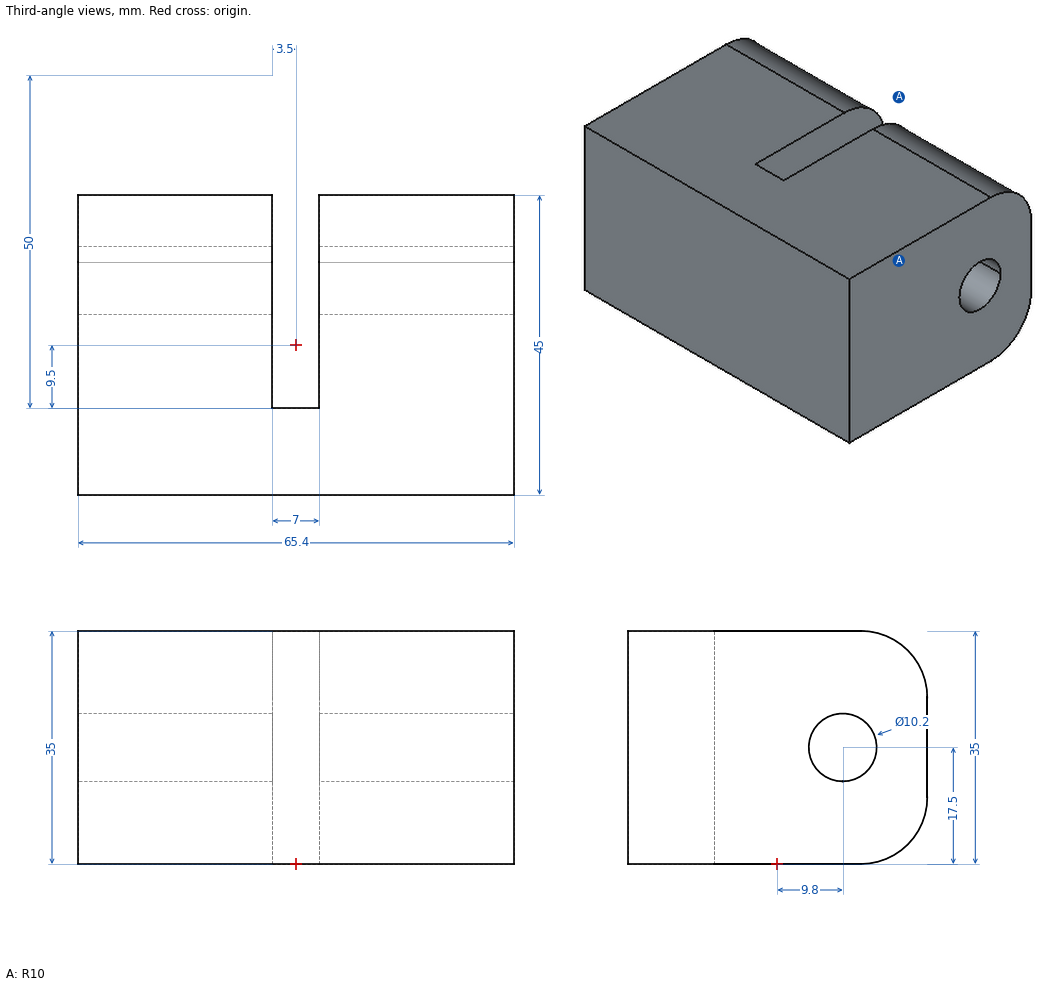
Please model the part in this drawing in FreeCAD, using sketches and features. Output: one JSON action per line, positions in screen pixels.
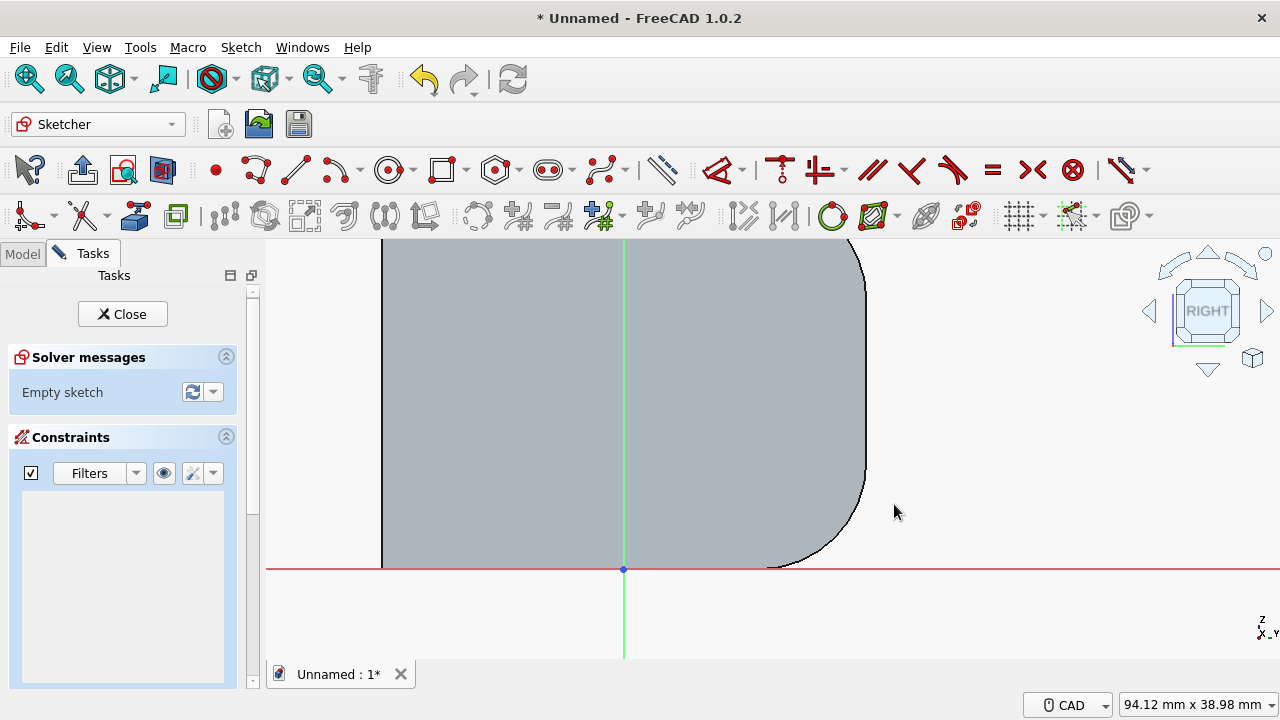
{"action": "left_click", "coordinate": [390, 170]}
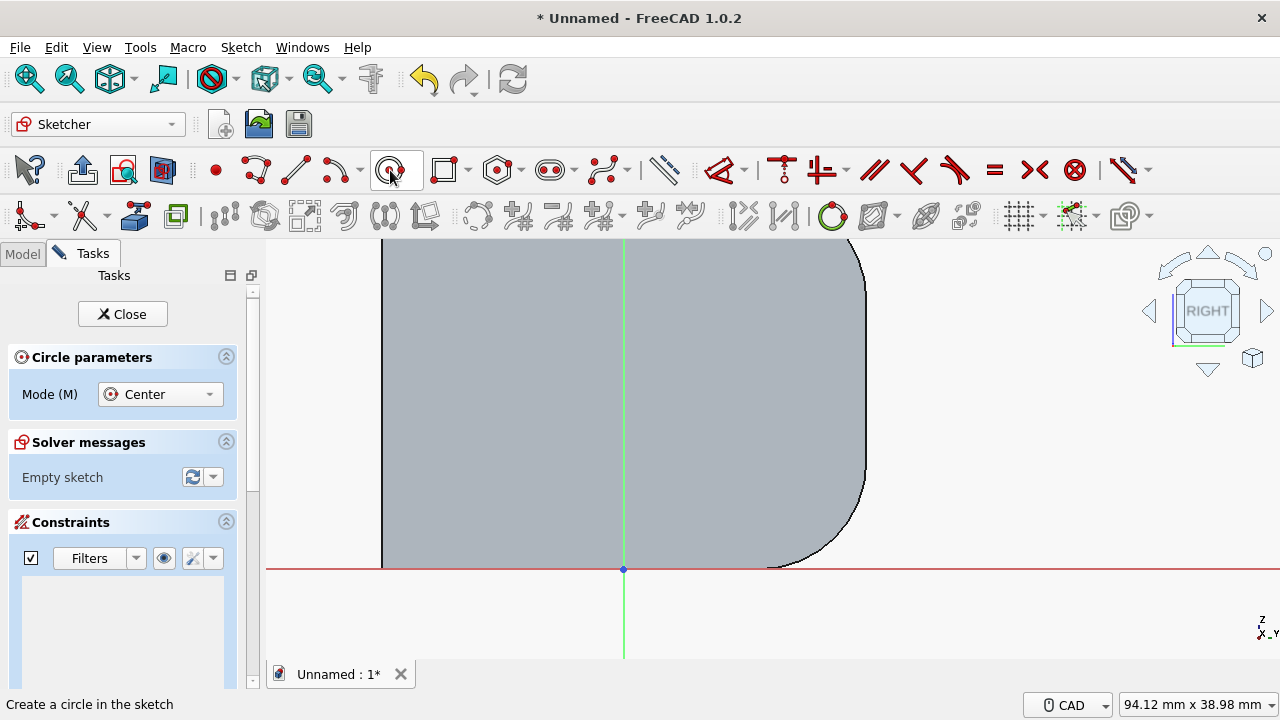
{"action": "left_click", "coordinate": [730, 381]}
{"action": "left_click", "coordinate": [768, 342]}
{"action": "key", "text": "Escape"}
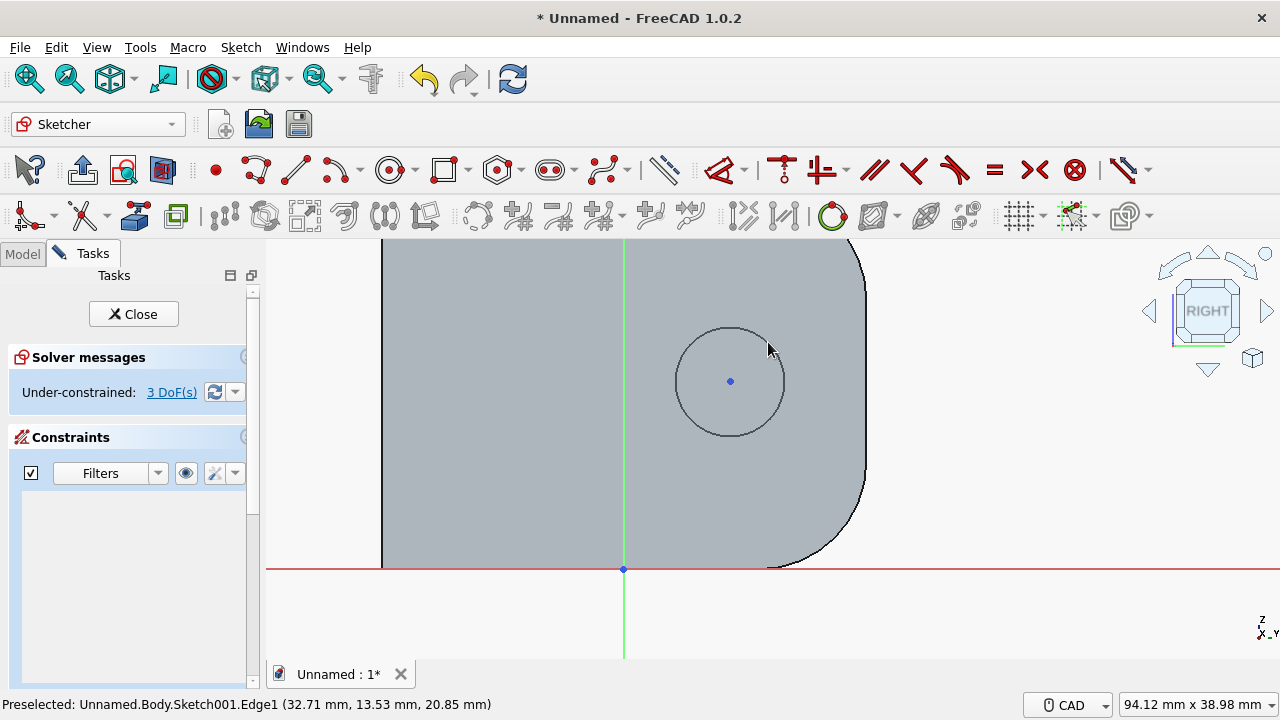
{"action": "left_click", "coordinate": [720, 170]}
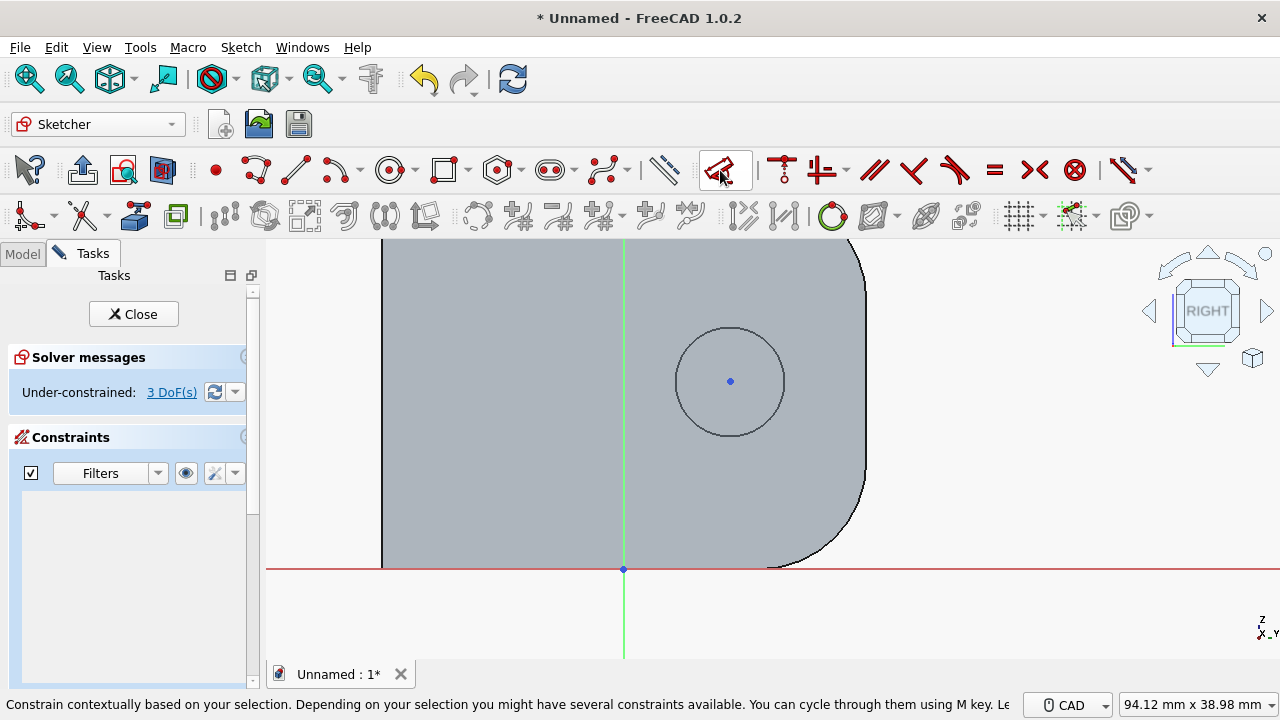
{"action": "left_click", "coordinate": [768, 343]}
{"action": "left_click", "coordinate": [790, 320]}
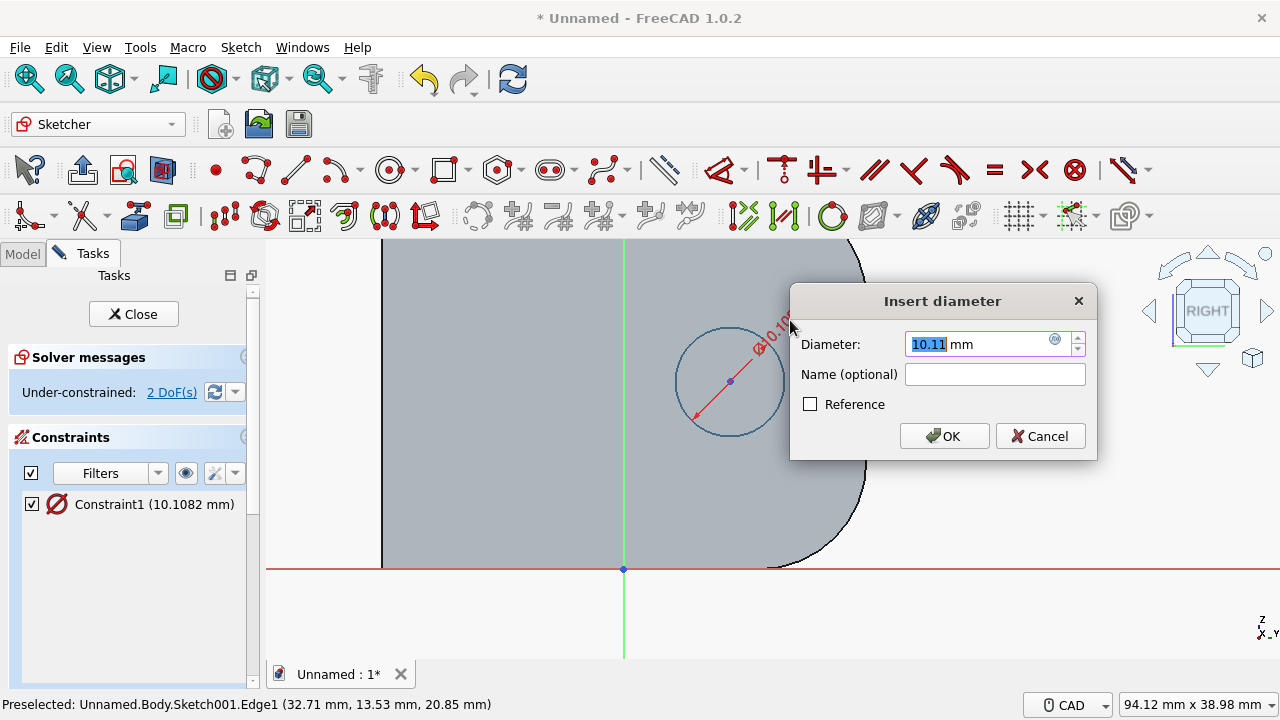
{"action": "type", "text": "10.2"}
{"action": "key", "text": "Return"}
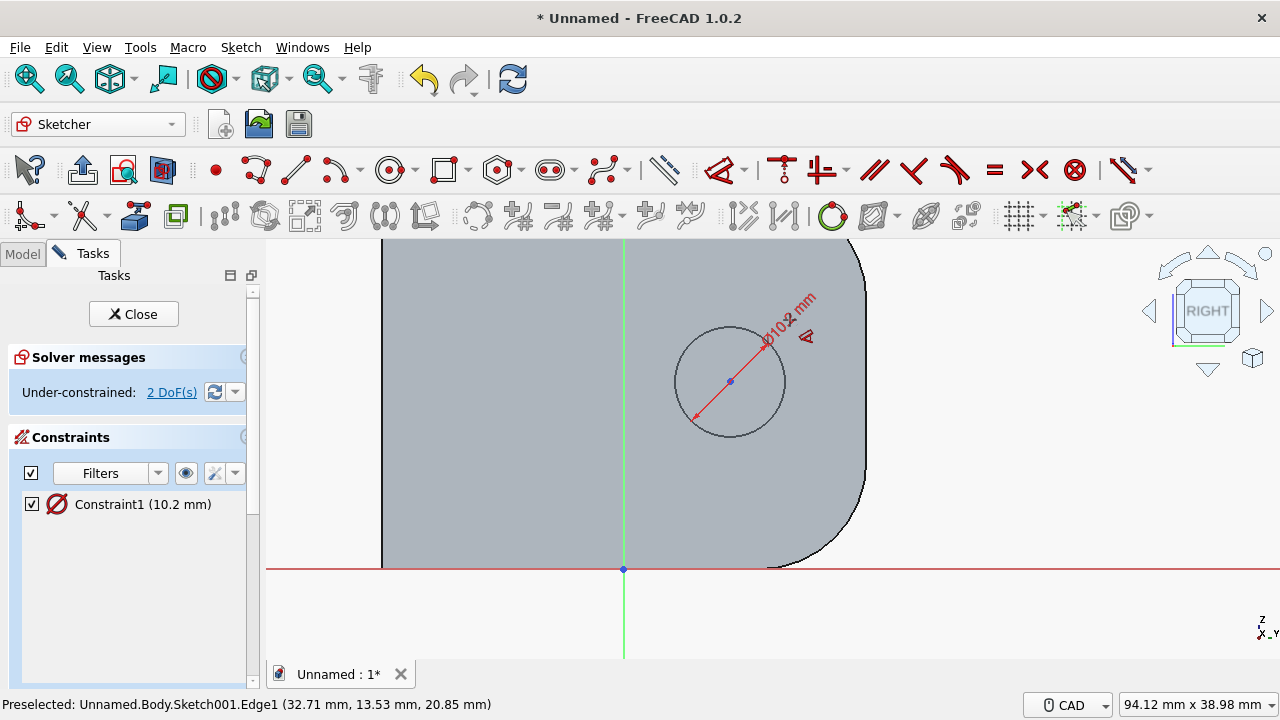
{"action": "left_click", "coordinate": [730, 382]}
{"action": "left_click", "coordinate": [677, 603]}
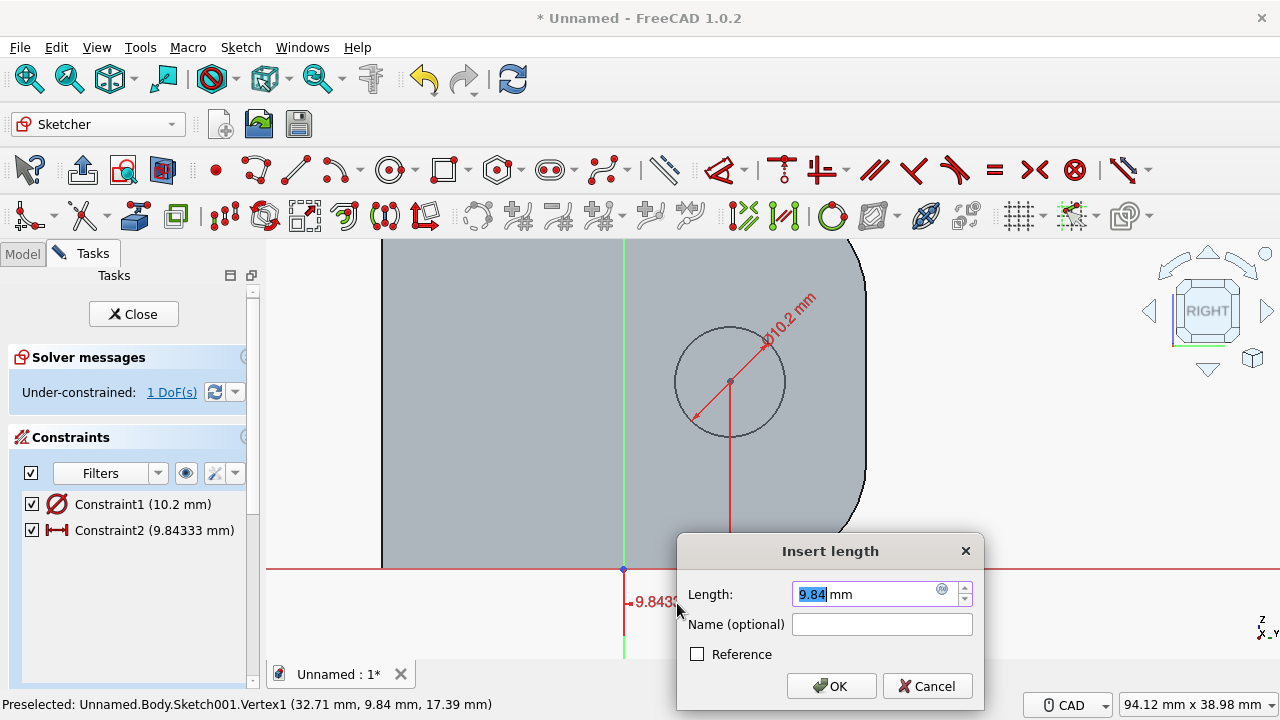
{"action": "type", "text": "9.8"}
{"action": "key", "text": "Return"}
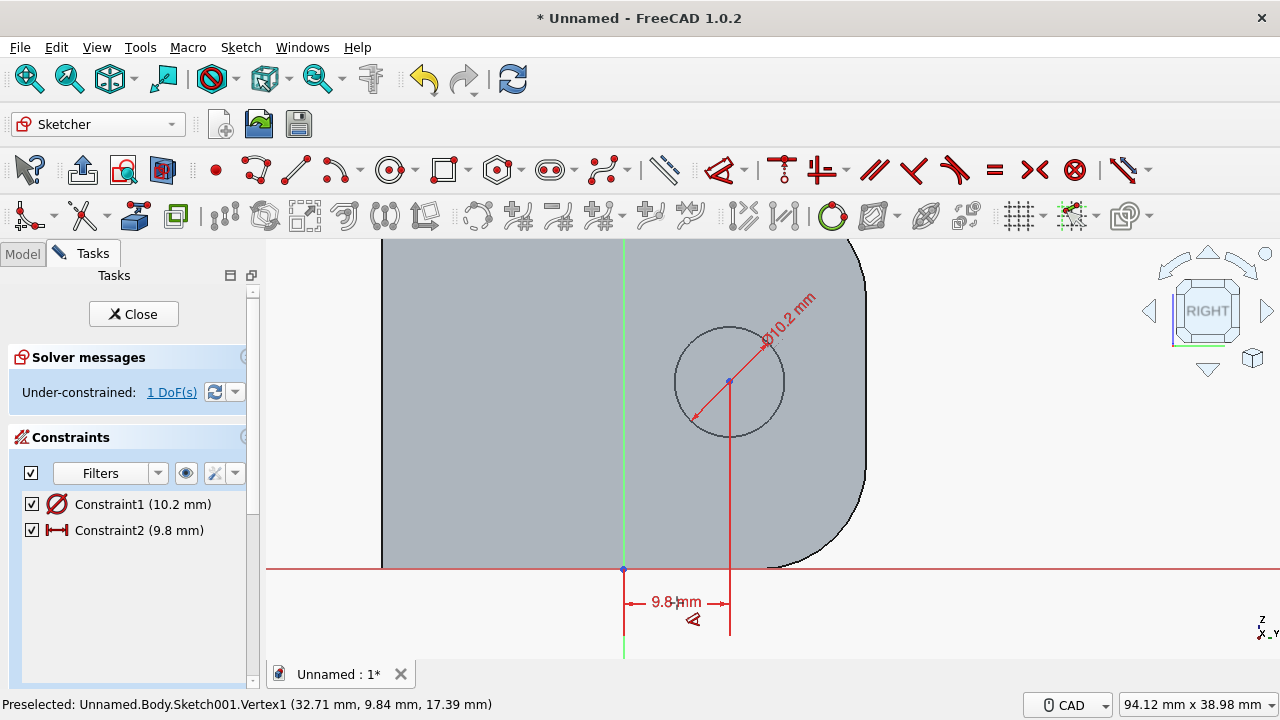
{"action": "left_click", "coordinate": [730, 382]}
{"action": "left_click", "coordinate": [590, 476]}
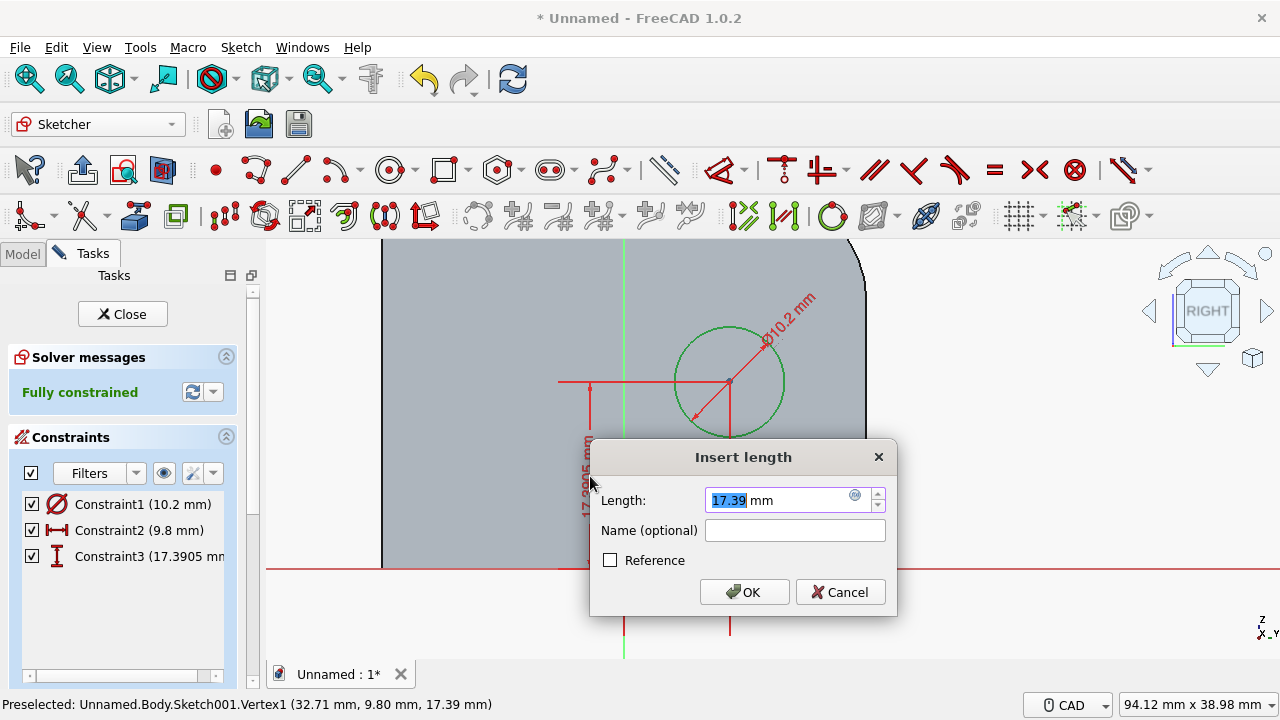
{"action": "type", "text": "17.5"}
{"action": "key", "text": "Return"}
{"action": "key", "text": "Escape"}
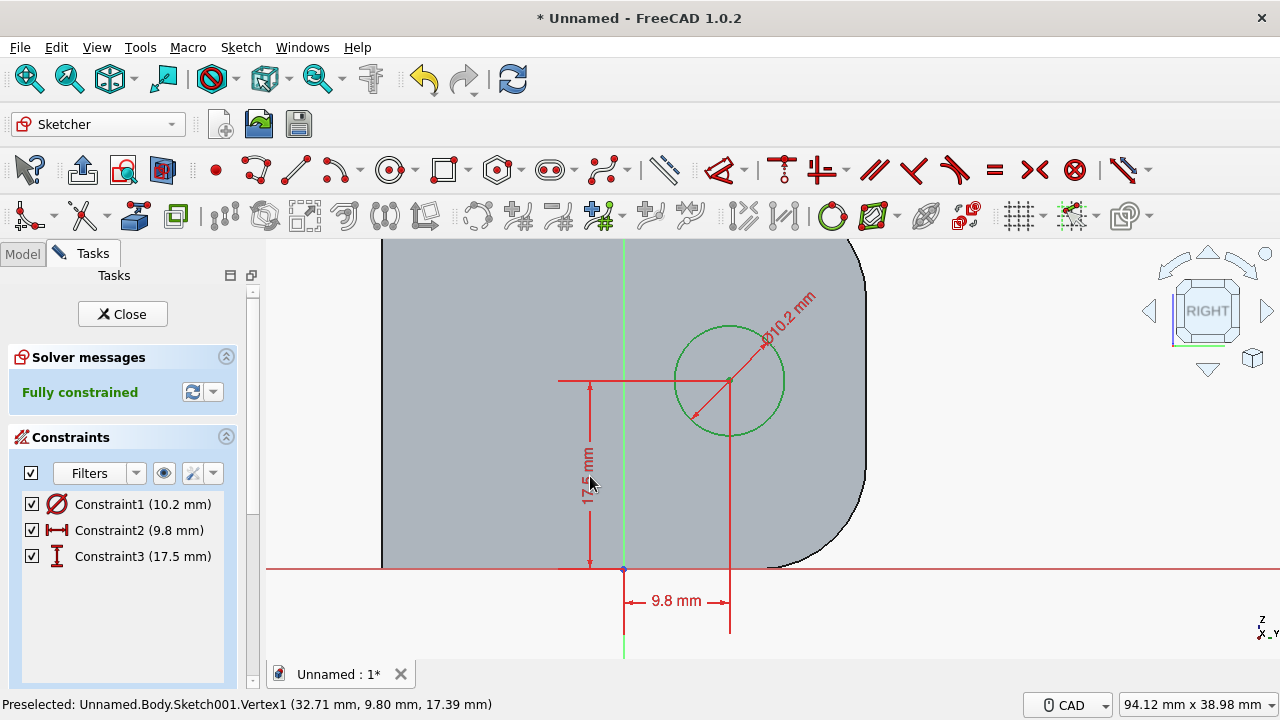
{"action": "left_click", "coordinate": [123, 314]}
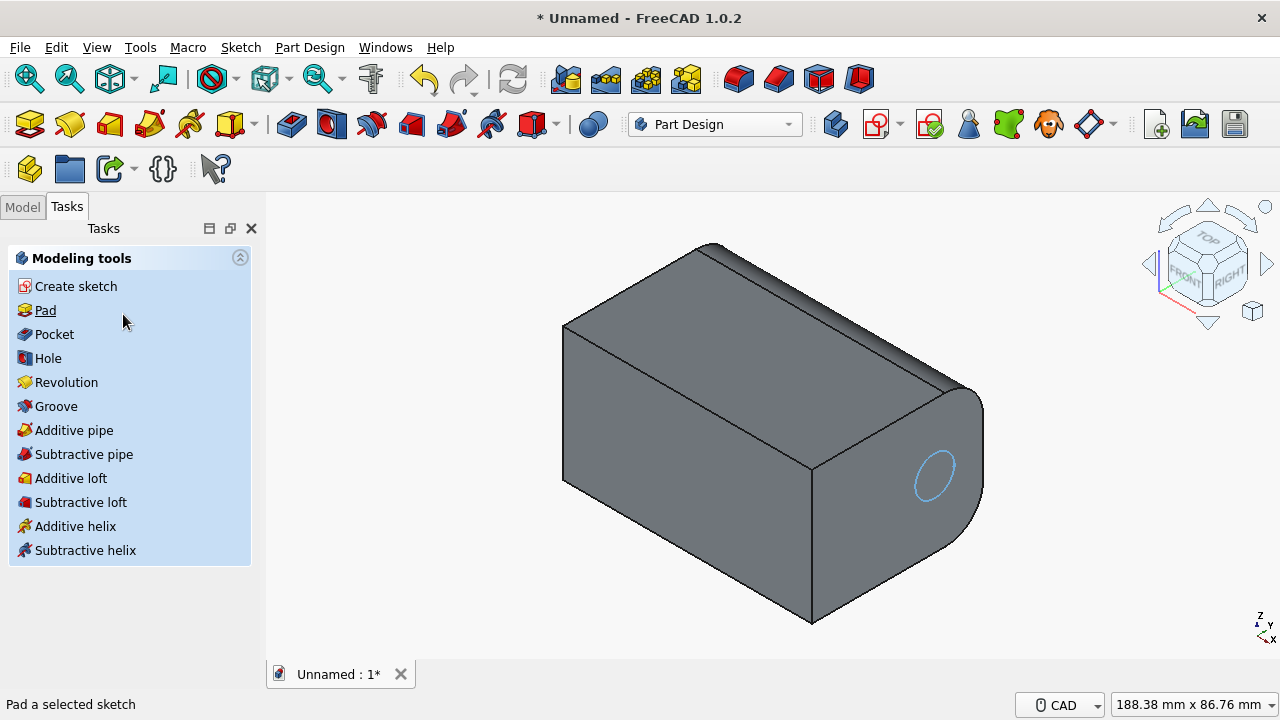
{"action": "left_click", "coordinate": [292, 124]}